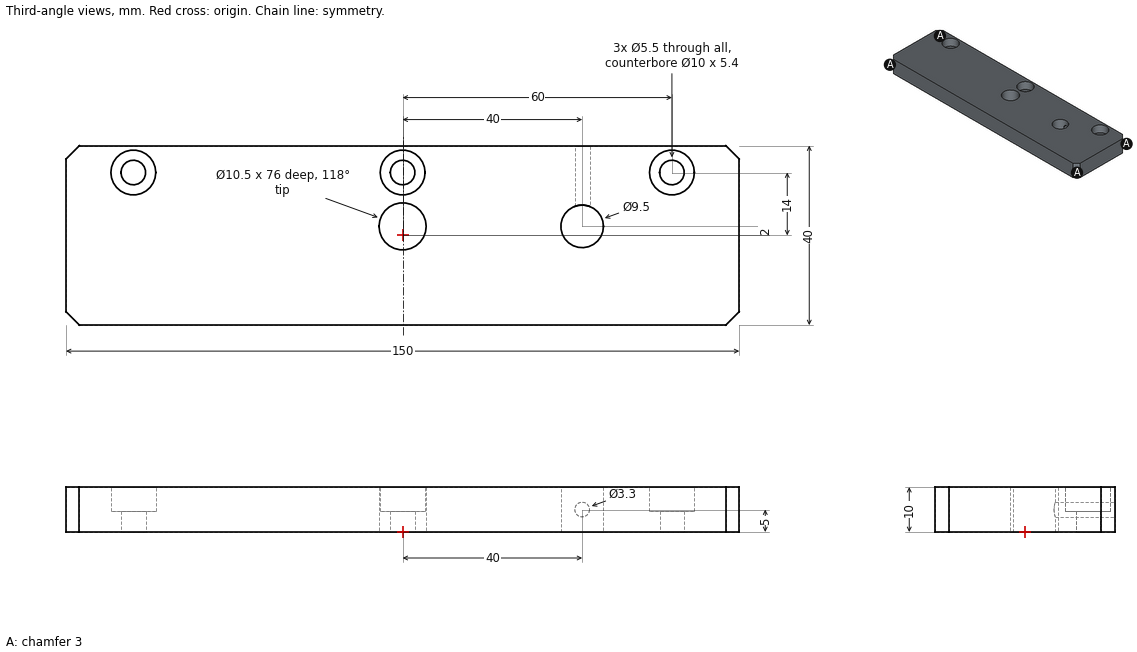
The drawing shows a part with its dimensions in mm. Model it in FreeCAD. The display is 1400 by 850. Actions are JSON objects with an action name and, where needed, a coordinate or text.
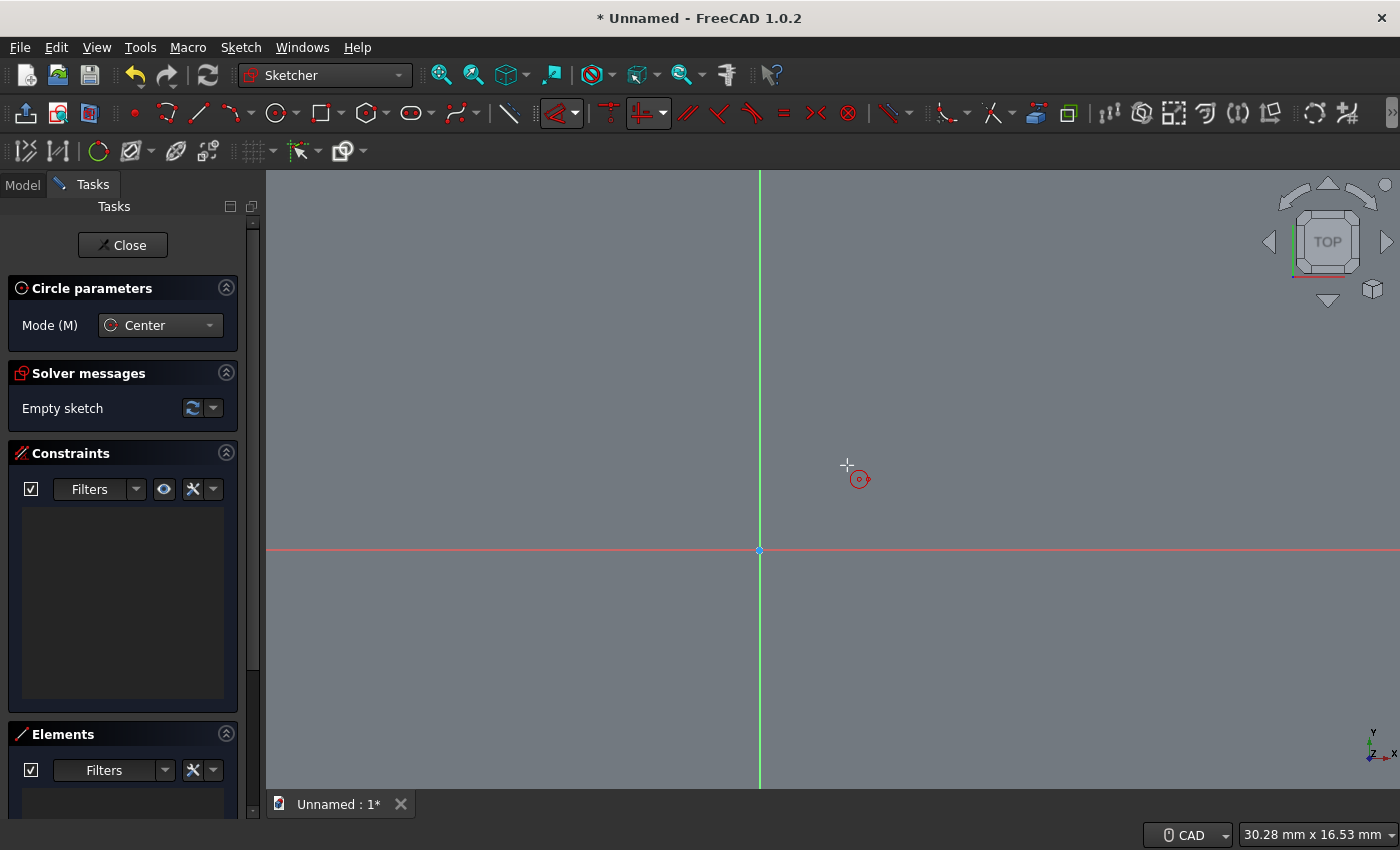
{"action": "left_click", "coordinate": [760, 475]}
{"action": "mouse_move", "coordinate": [899, 336]}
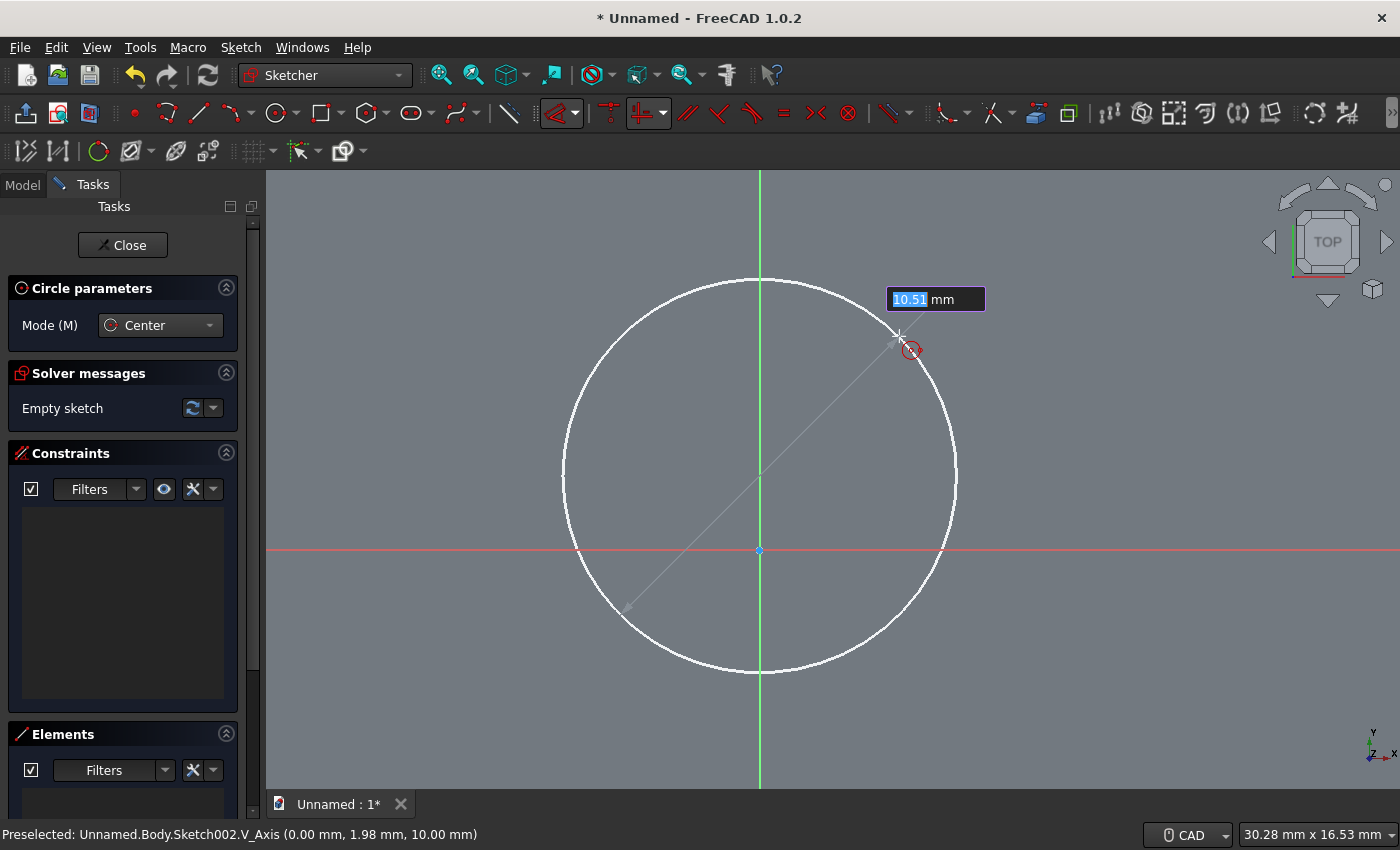
{"action": "type", "text": "10.5"}
{"action": "key", "text": "Return"}
{"action": "key", "text": "Escape"}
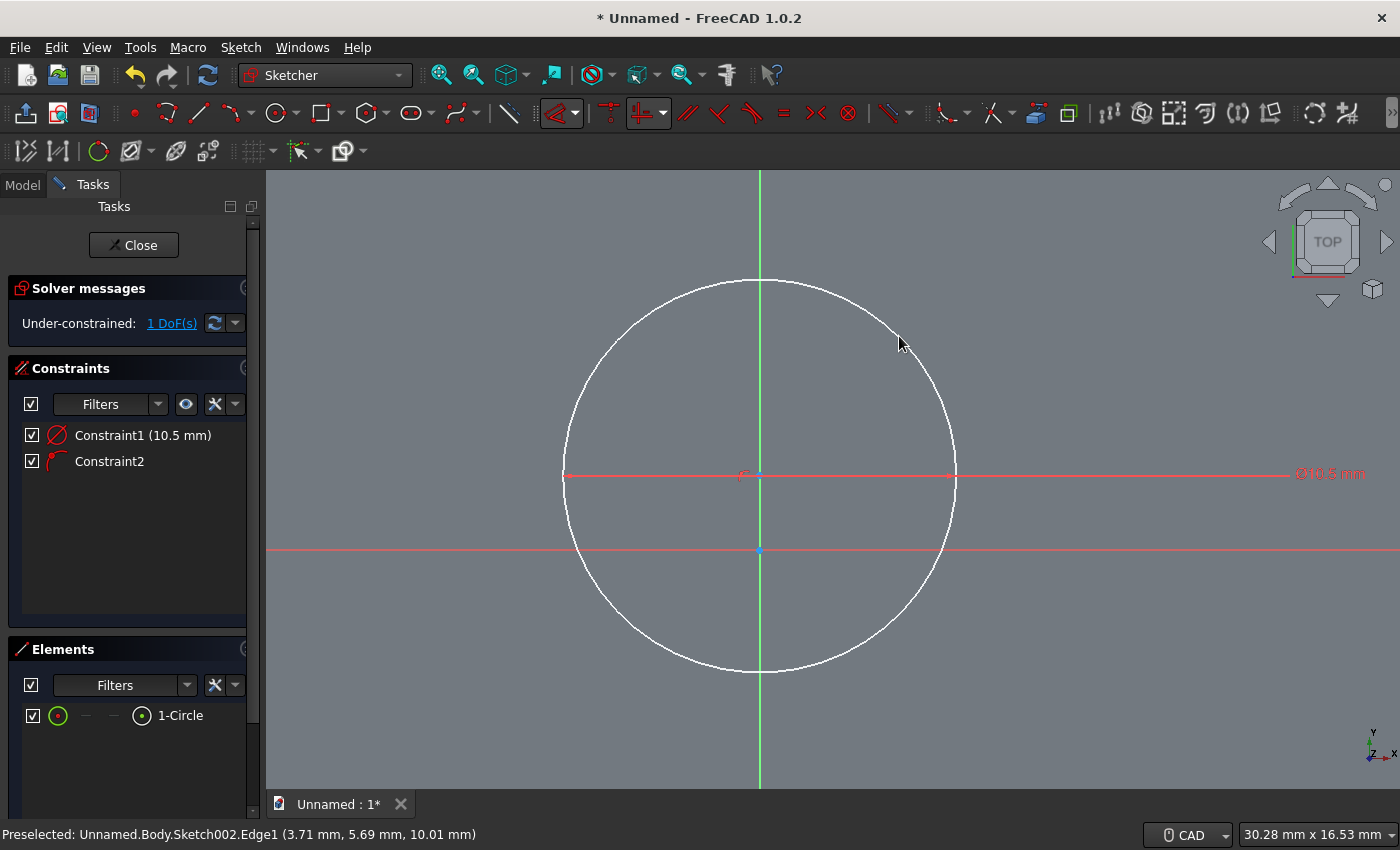
{"action": "left_click", "coordinate": [556, 114]}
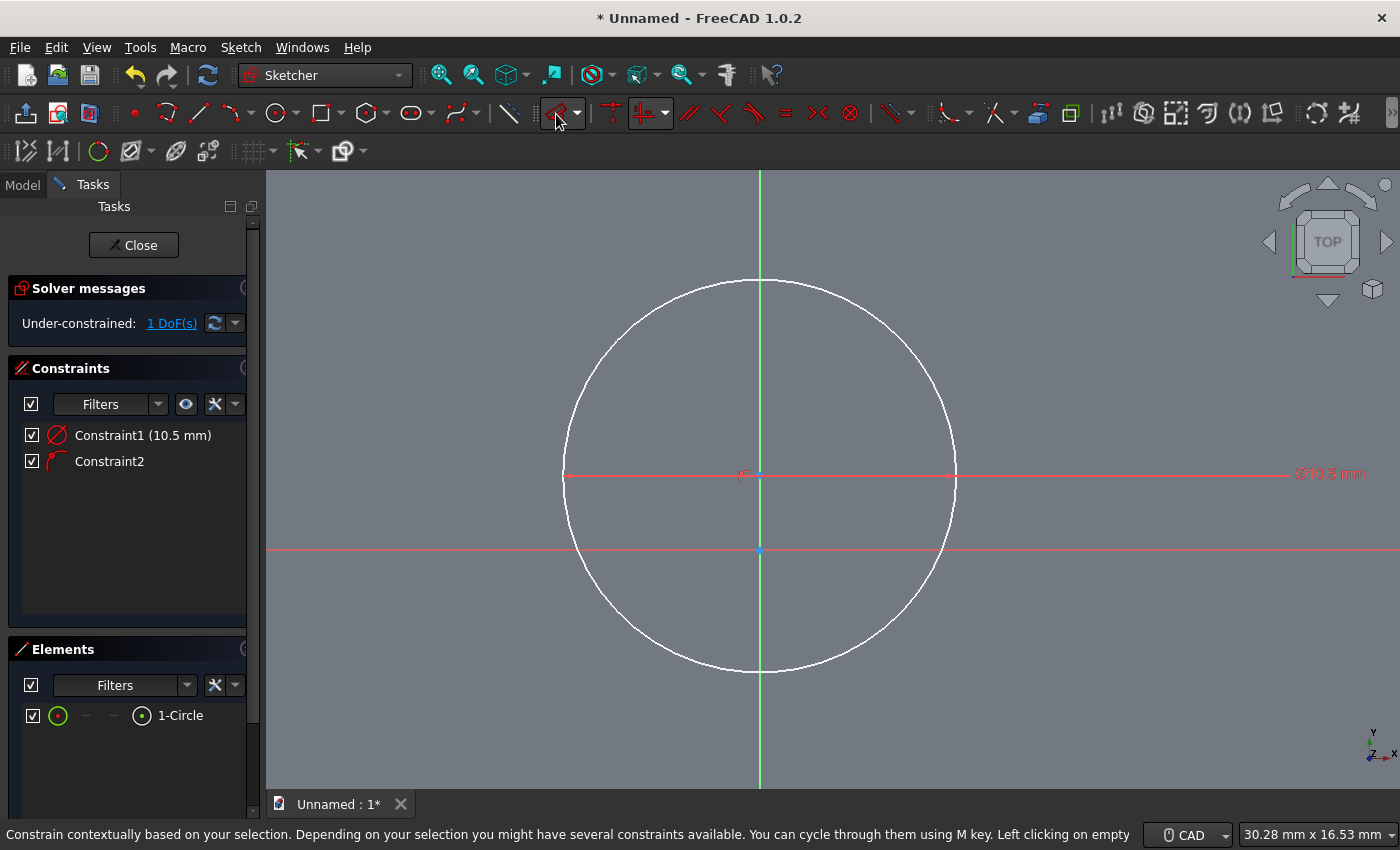
{"action": "left_click", "coordinate": [760, 476]}
{"action": "left_click", "coordinate": [794, 513]}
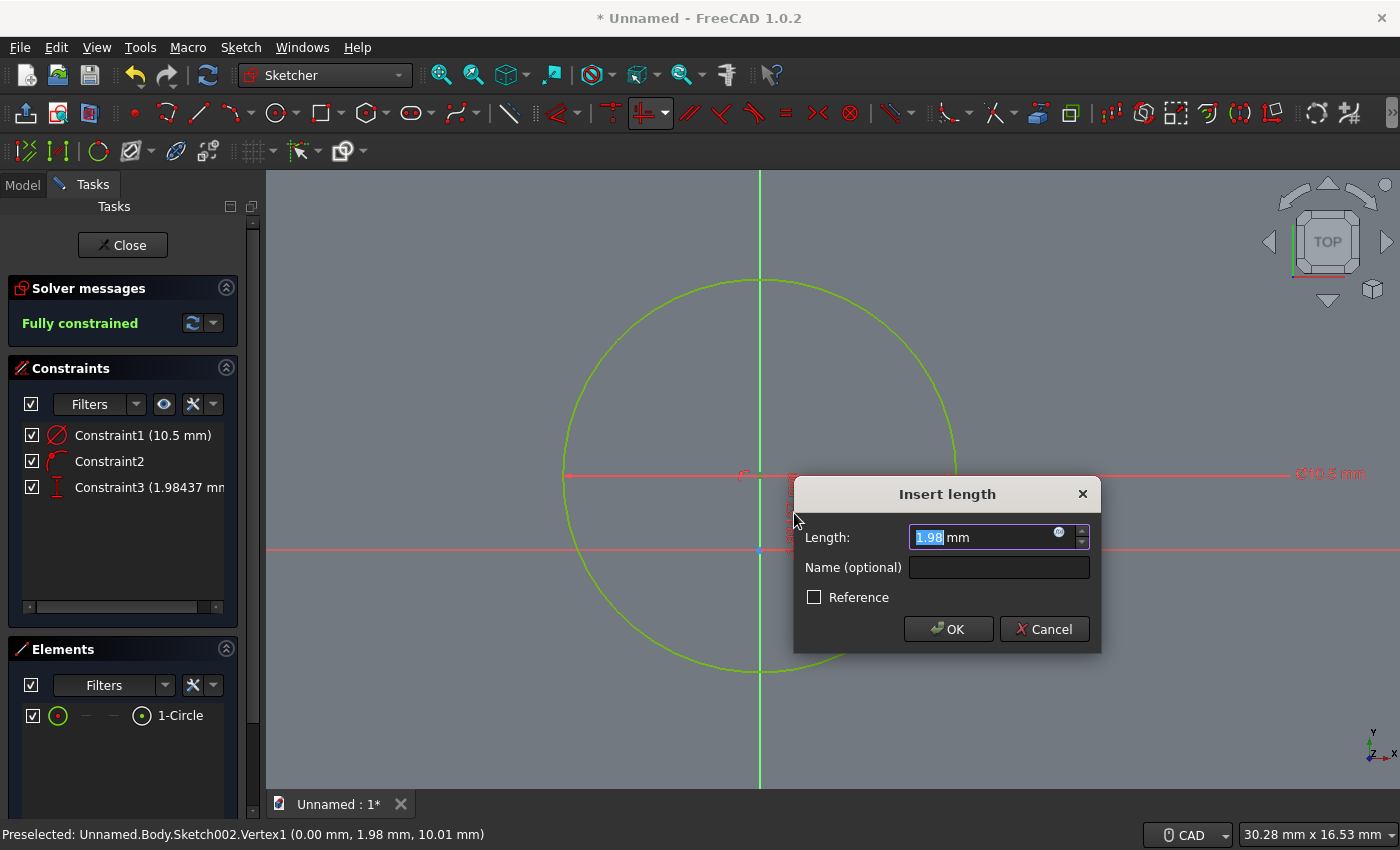
{"action": "type", "text": "2"}
{"action": "key", "text": "Return"}
{"action": "key", "text": "Escape"}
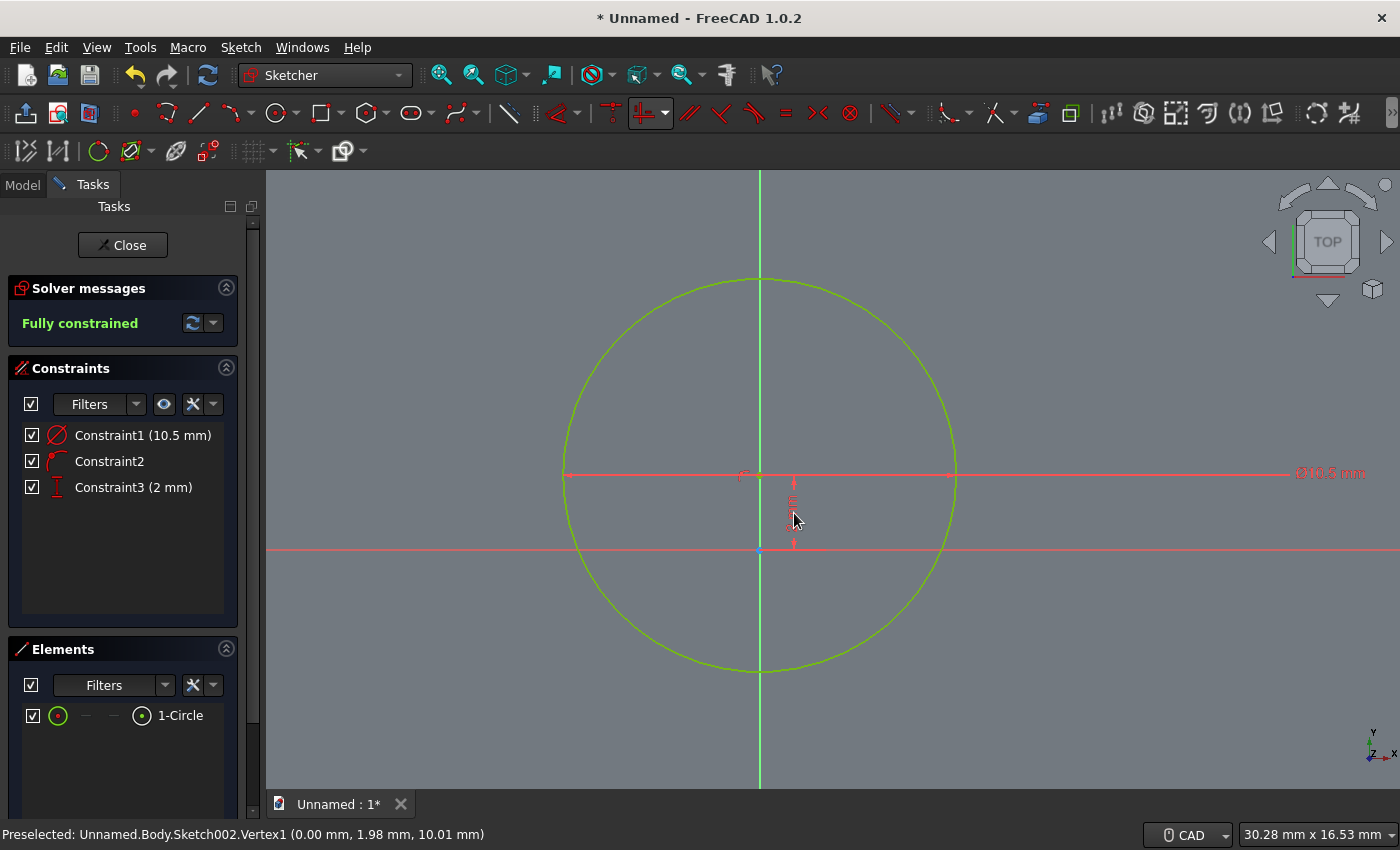
{"action": "left_click", "coordinate": [123, 245]}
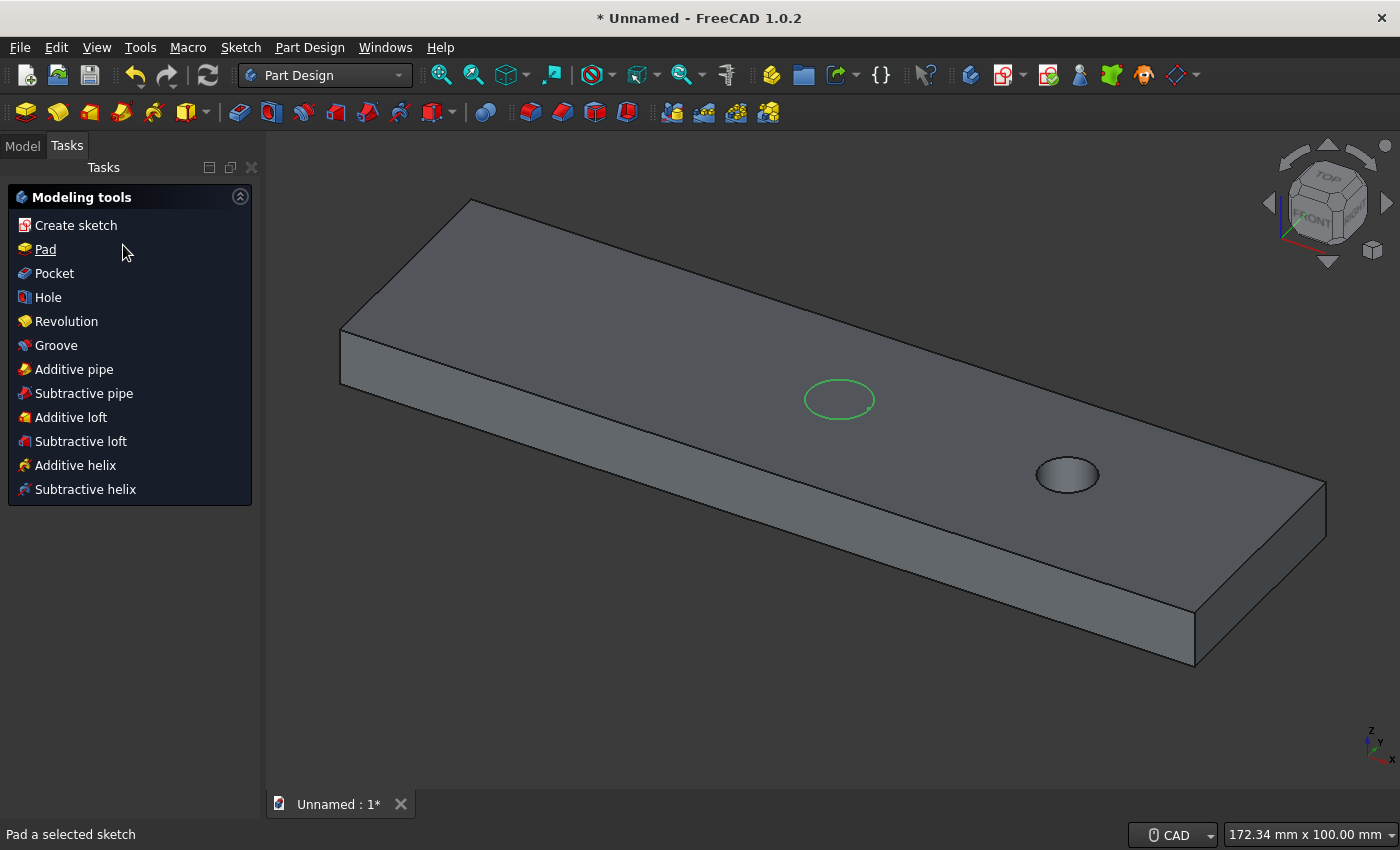
{"action": "left_click", "coordinate": [272, 112]}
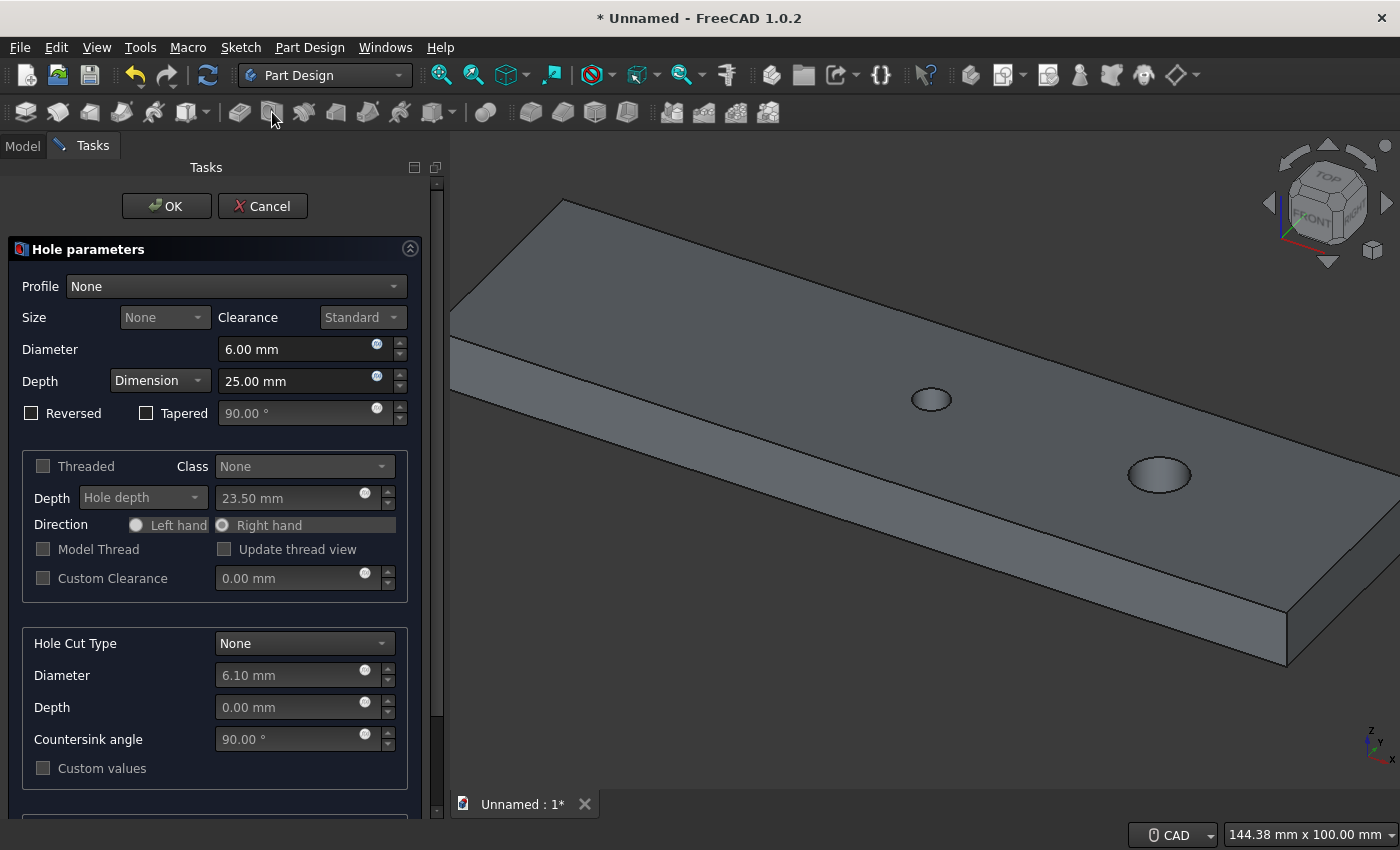
{"action": "triple_click", "coordinate": [305, 349]}